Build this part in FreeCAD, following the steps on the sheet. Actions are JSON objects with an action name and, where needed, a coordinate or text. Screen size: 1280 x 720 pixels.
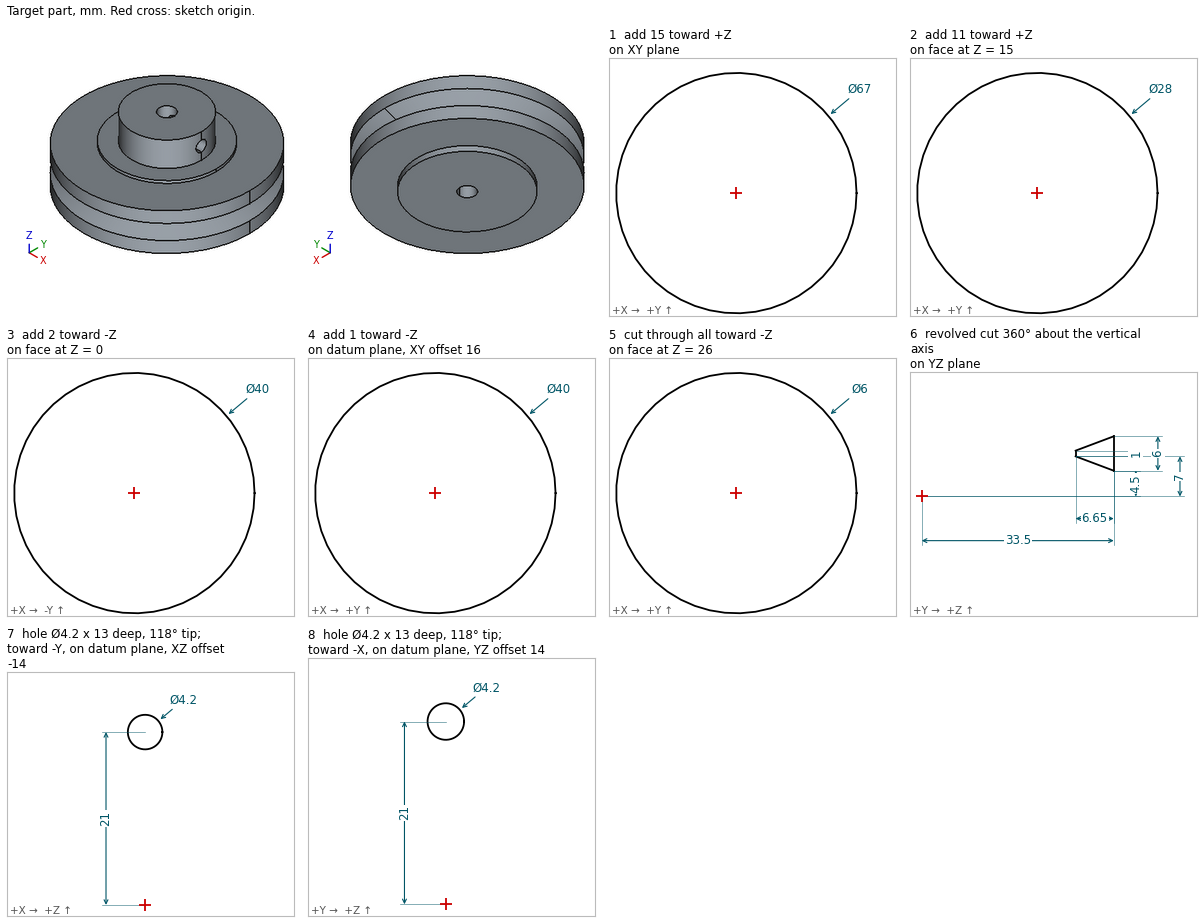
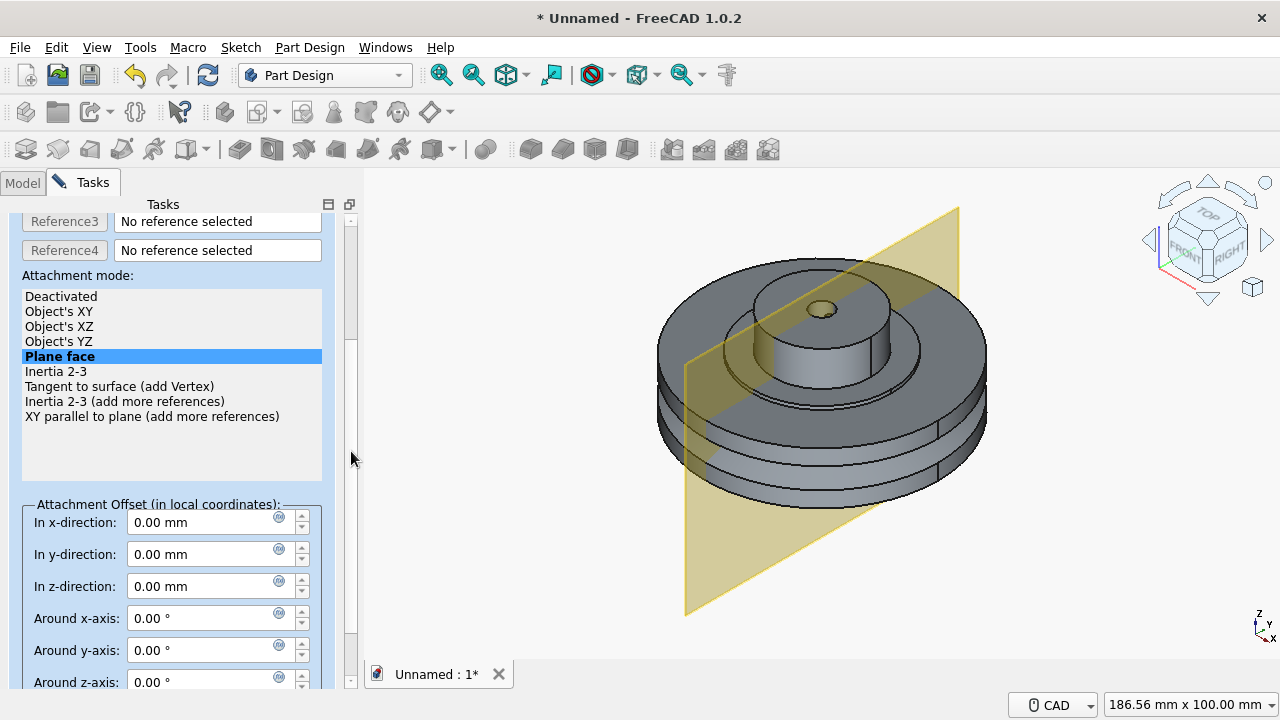
{"action": "triple_click", "coordinate": [210, 586]}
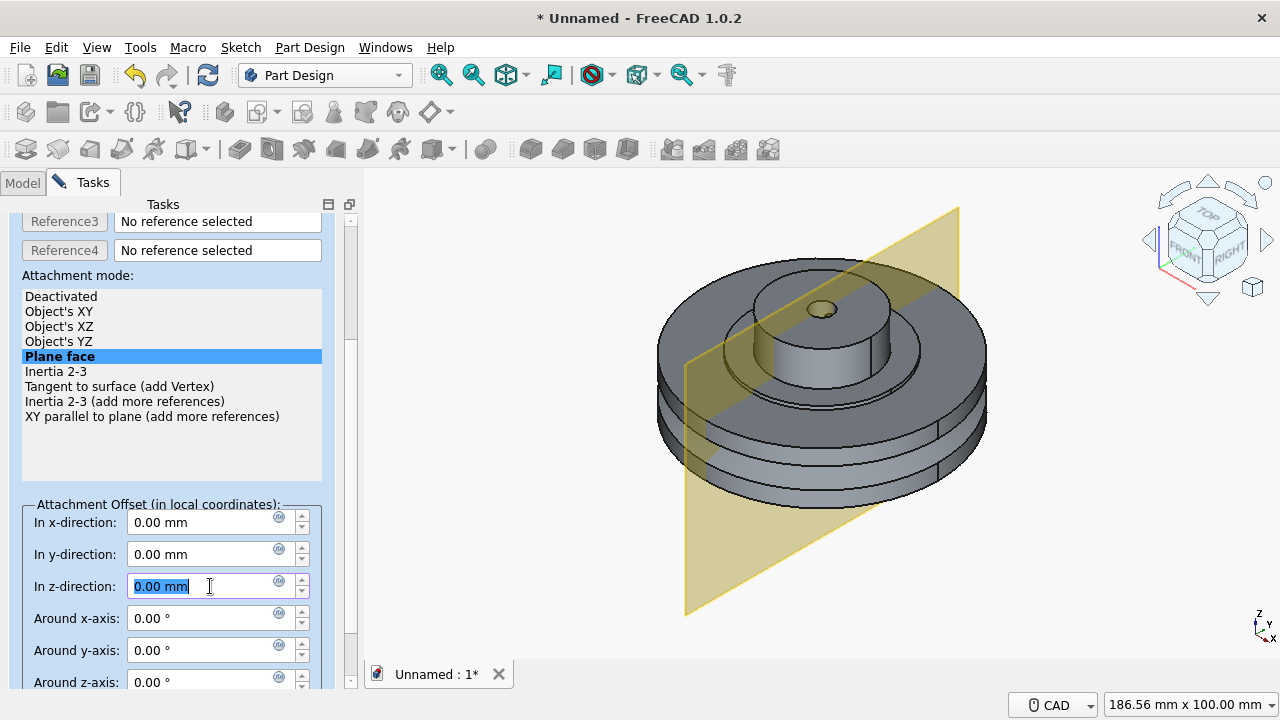
{"action": "type", "text": "14"}
{"action": "key", "text": "Tab"}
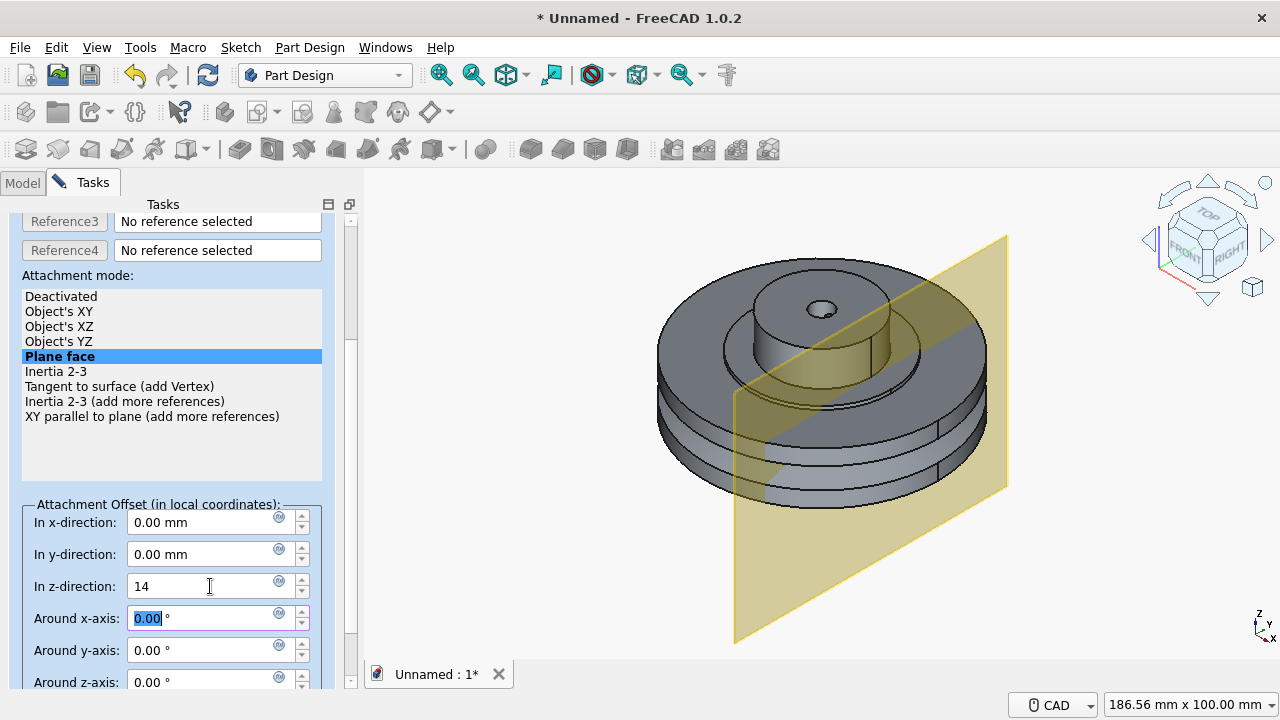
{"action": "scroll", "coordinate": [351, 451], "scroll_direction": "up", "scroll_amount": 4}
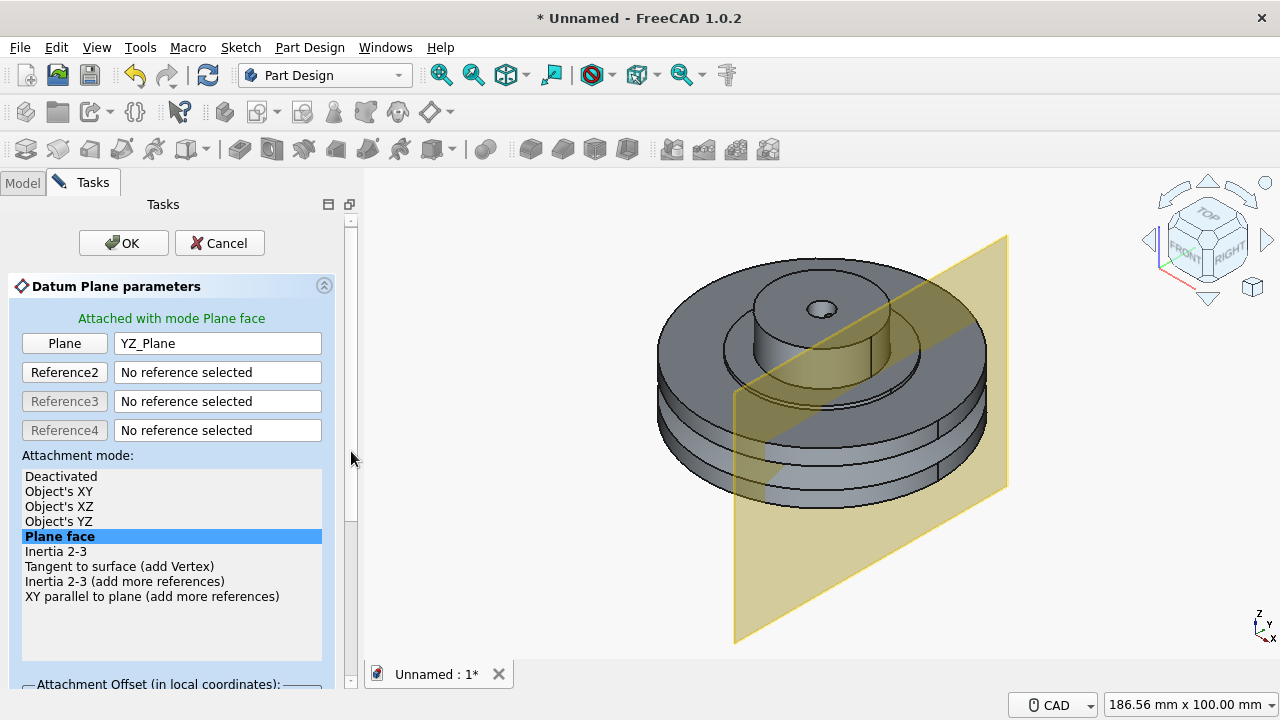
{"action": "left_click", "coordinate": [124, 243]}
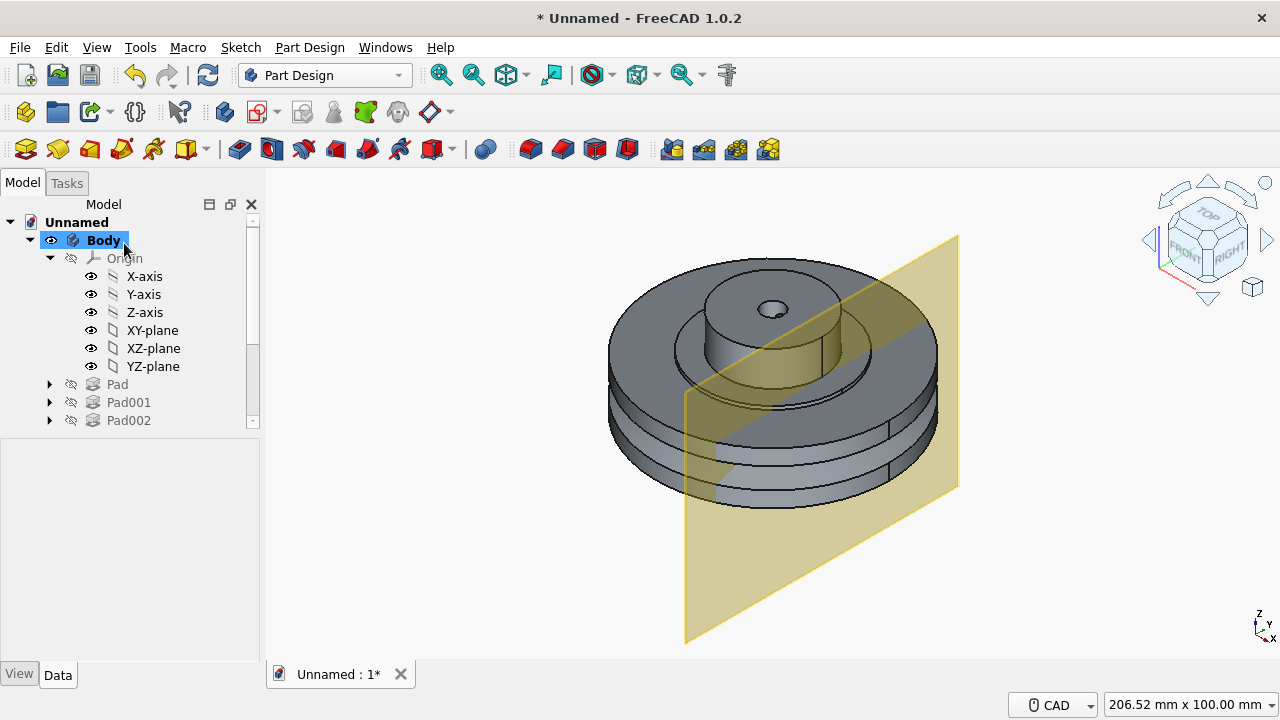
{"action": "scroll", "coordinate": [100, 326], "scroll_direction": "down", "scroll_amount": 3}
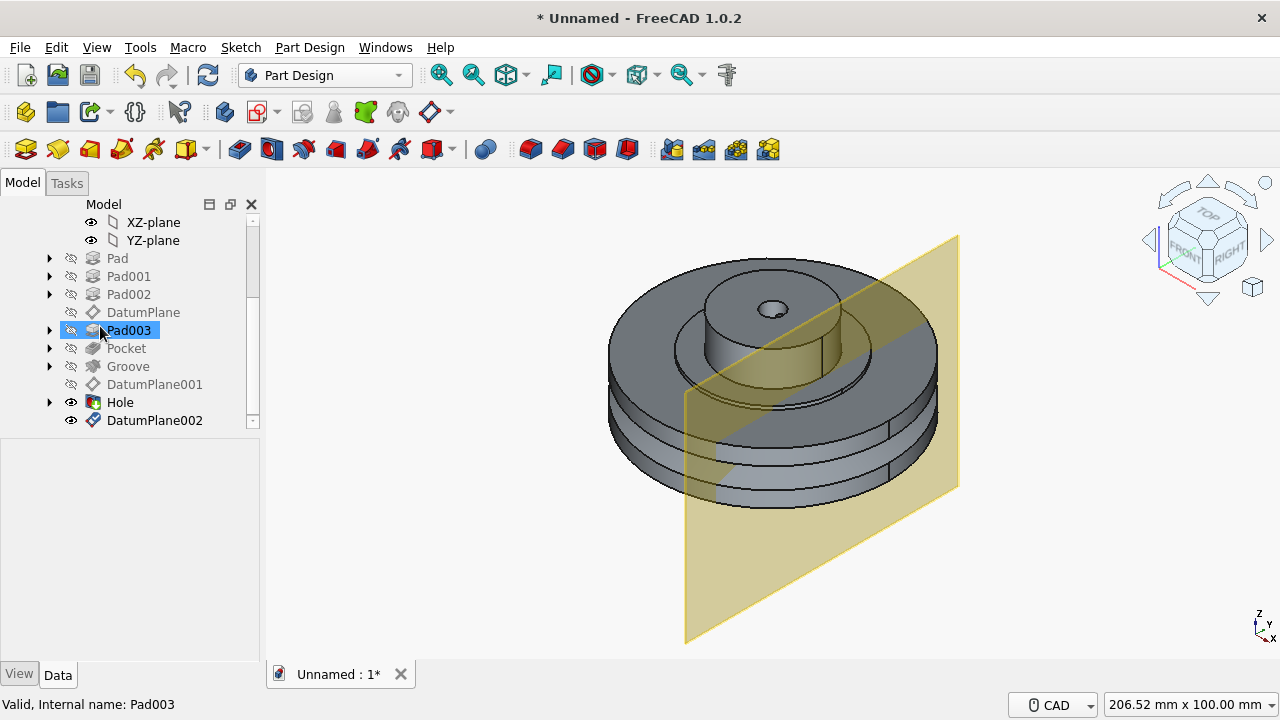
{"action": "left_click", "coordinate": [116, 420]}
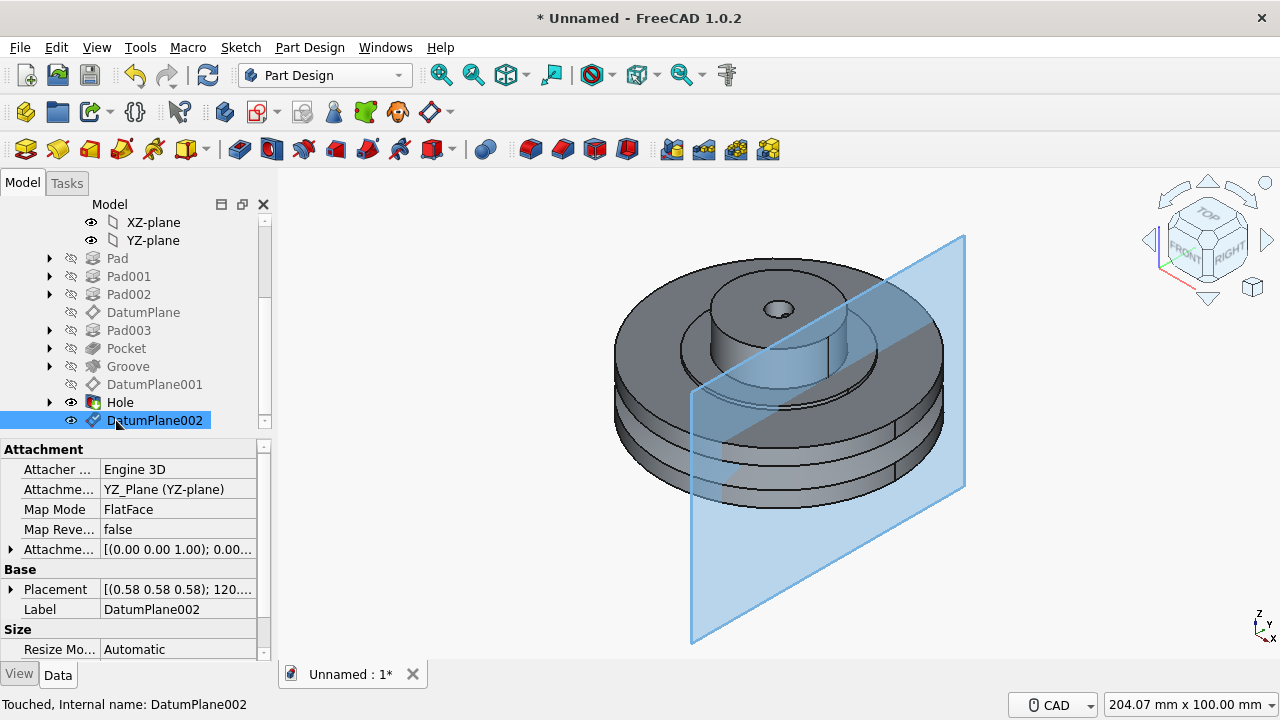
{"action": "left_click", "coordinate": [258, 112]}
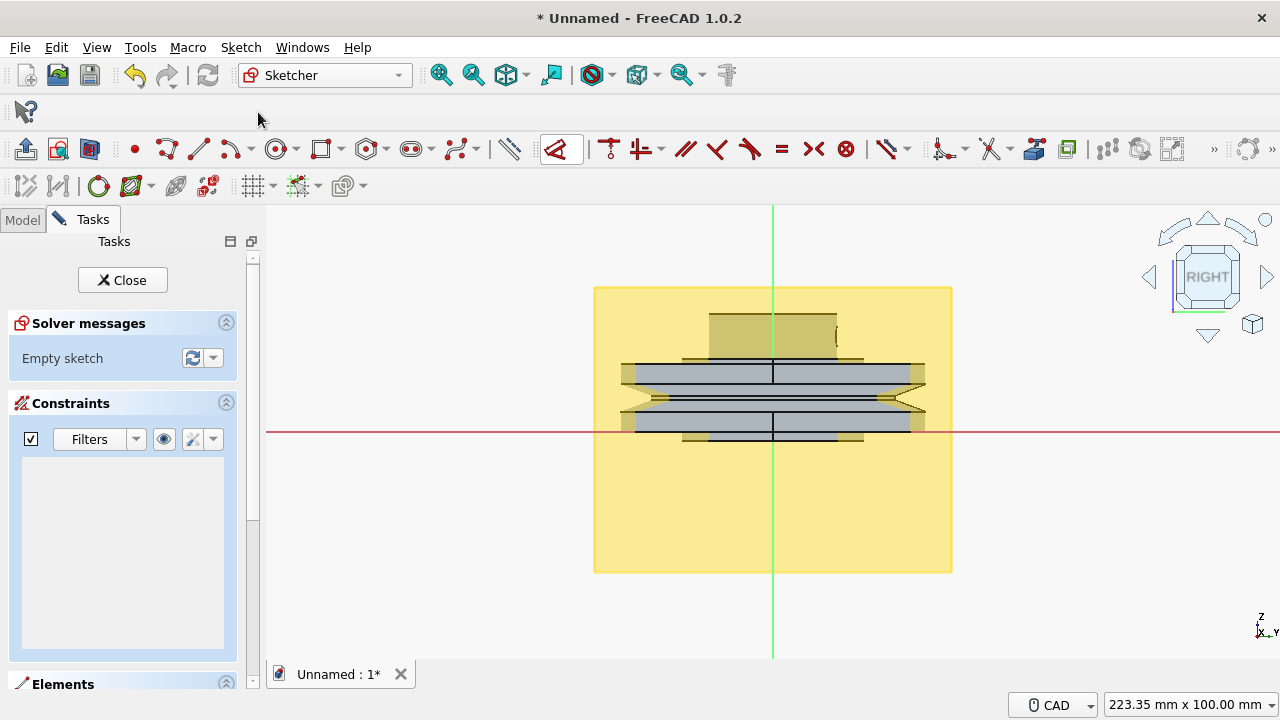
{"action": "key", "text": "q s"}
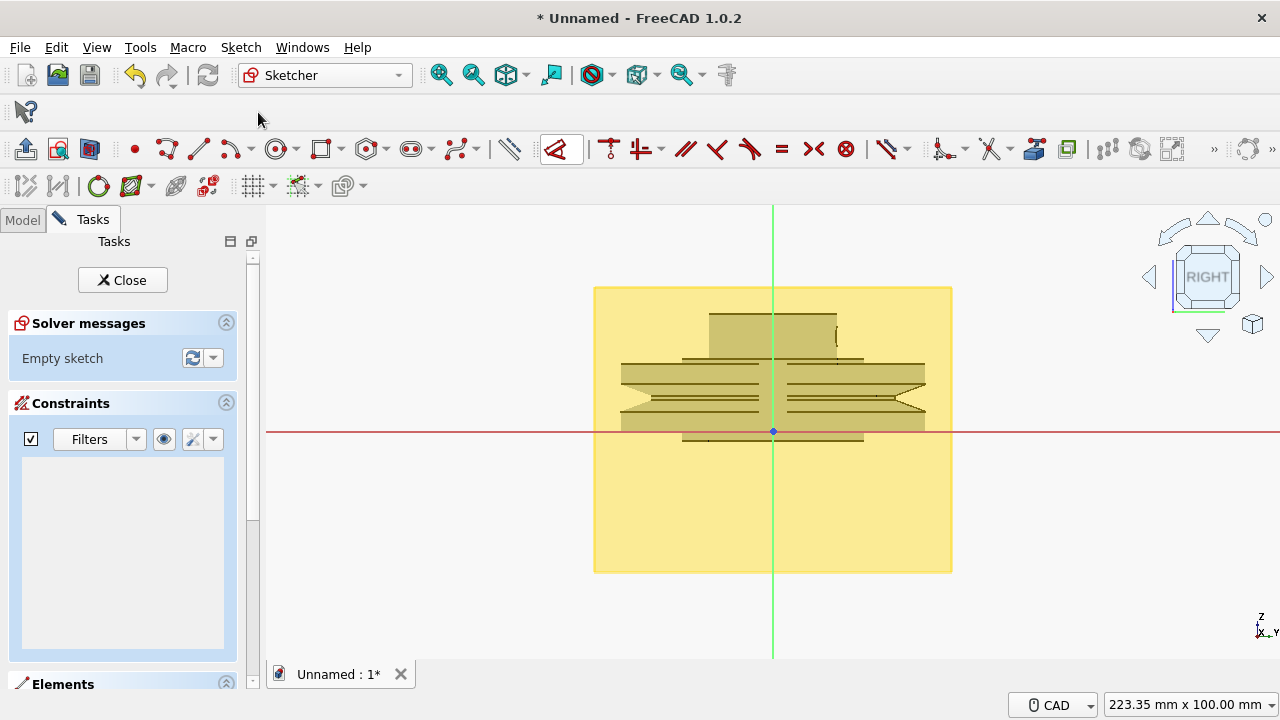
{"action": "scroll", "coordinate": [778, 329], "scroll_direction": "up", "scroll_amount": 13}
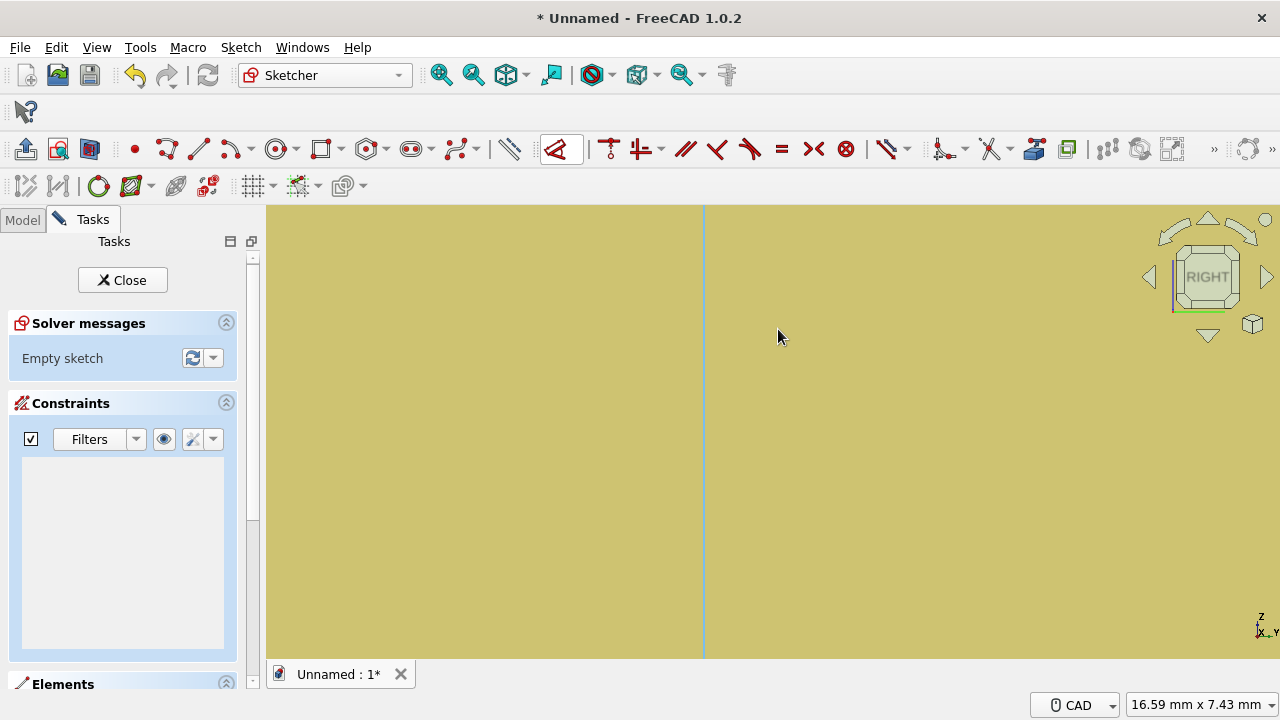
{"action": "key", "text": "g c"}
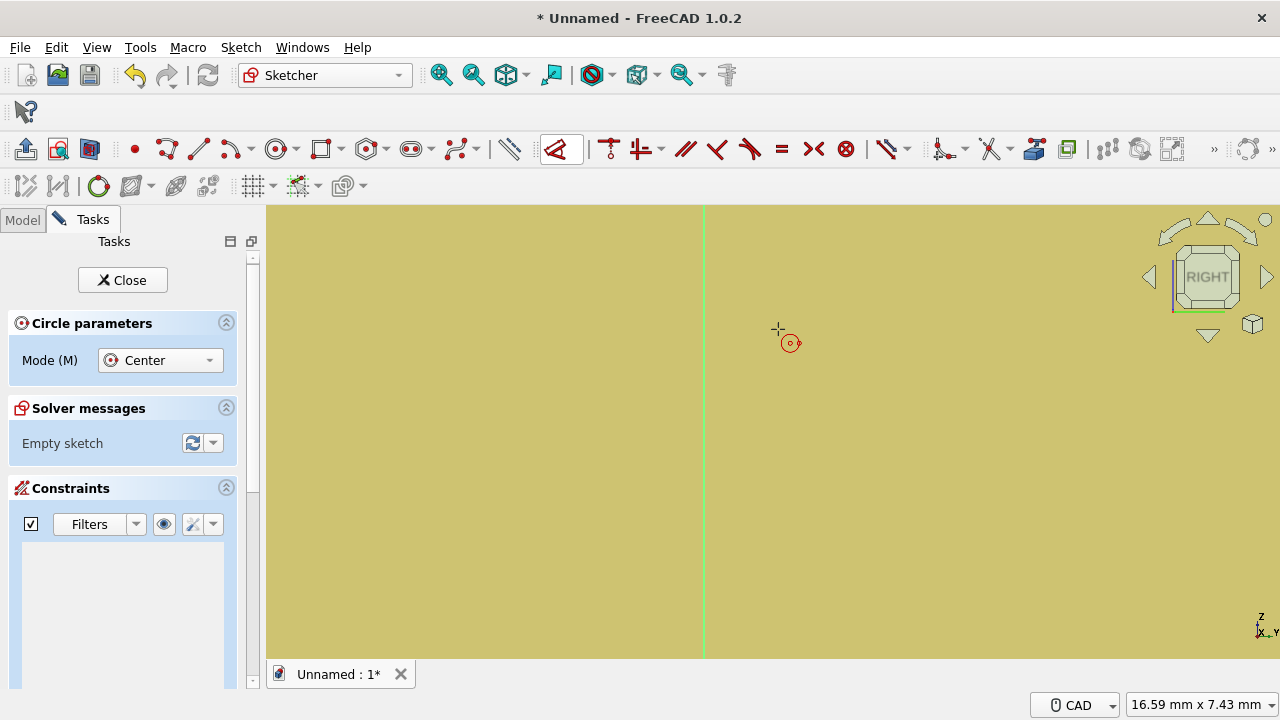
{"action": "left_click", "coordinate": [704, 429]}
{"action": "left_click", "coordinate": [795, 338]}
{"action": "key", "text": "Escape"}